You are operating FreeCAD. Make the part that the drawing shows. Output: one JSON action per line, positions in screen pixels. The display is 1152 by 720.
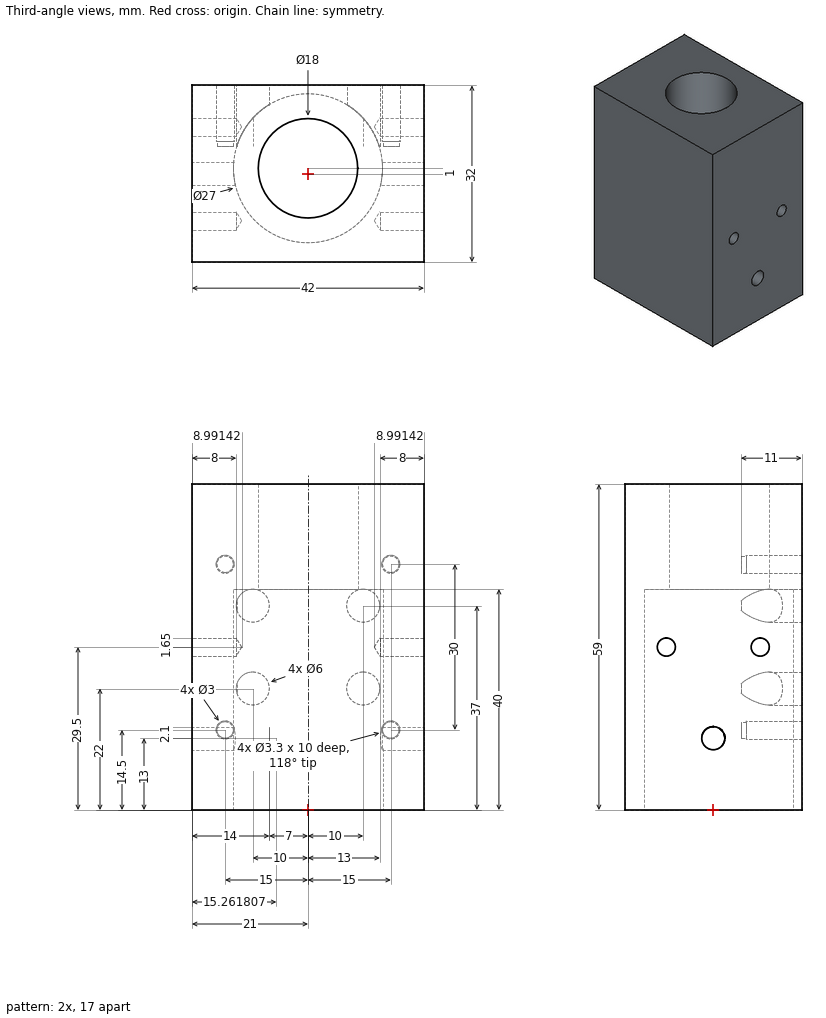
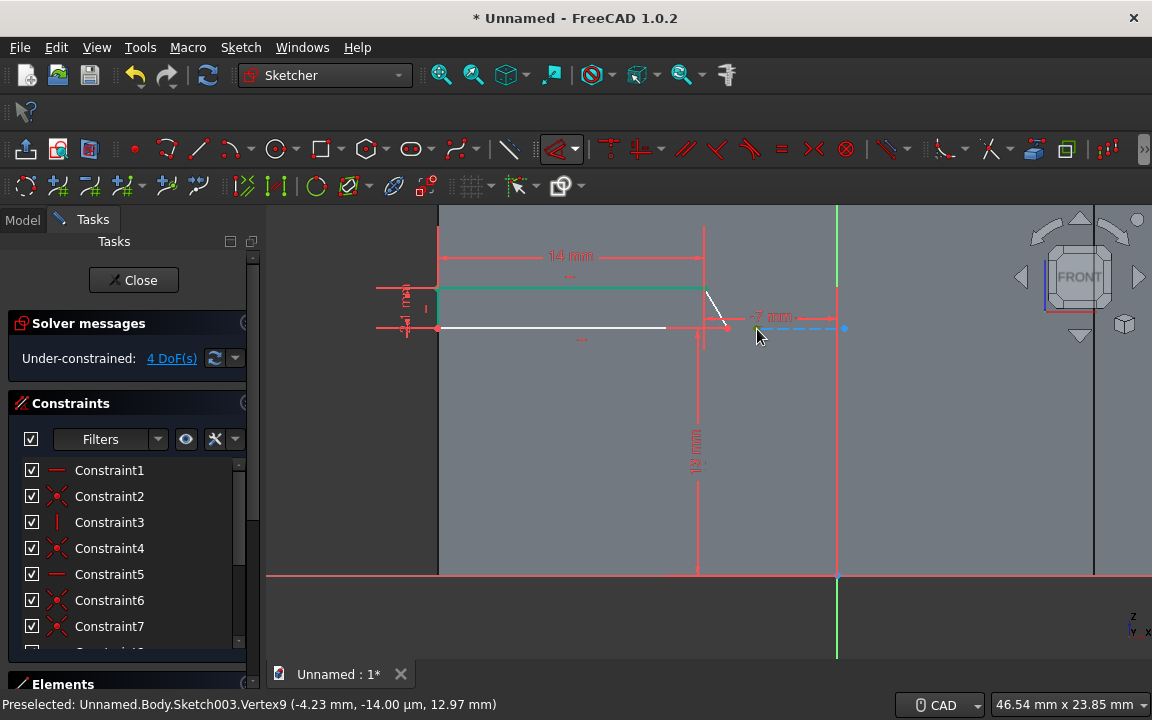
{"action": "key", "text": "i"}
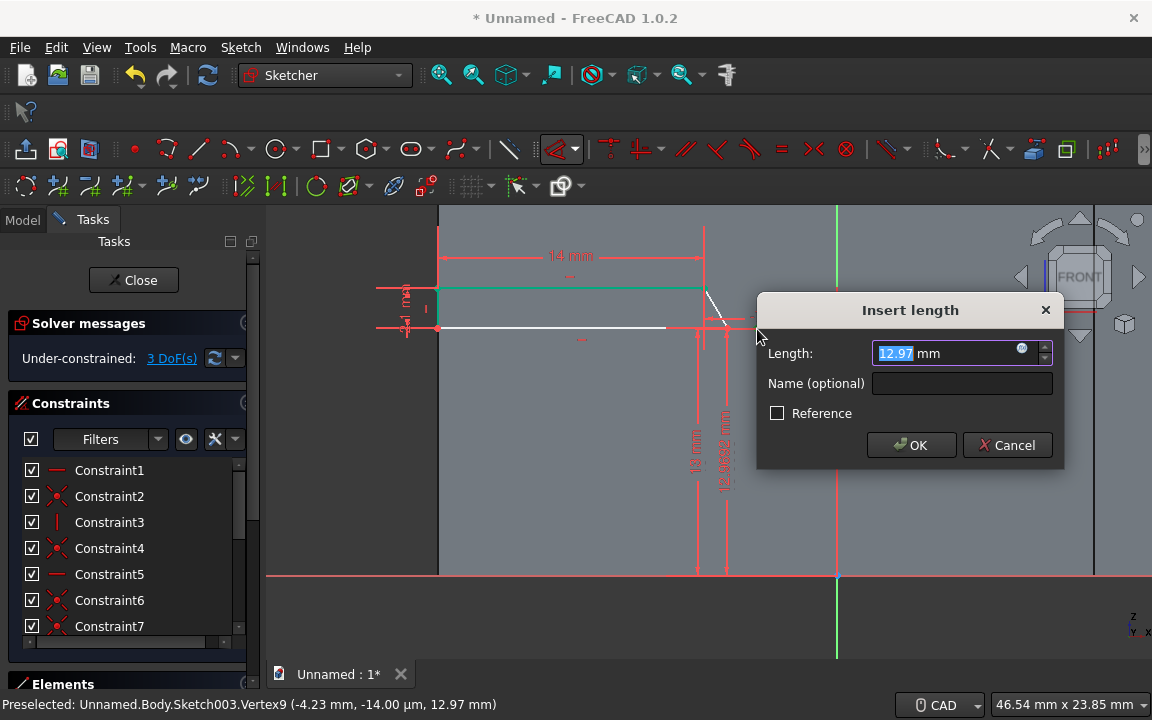
{"action": "type", "text": "13"}
{"action": "key", "text": "Return"}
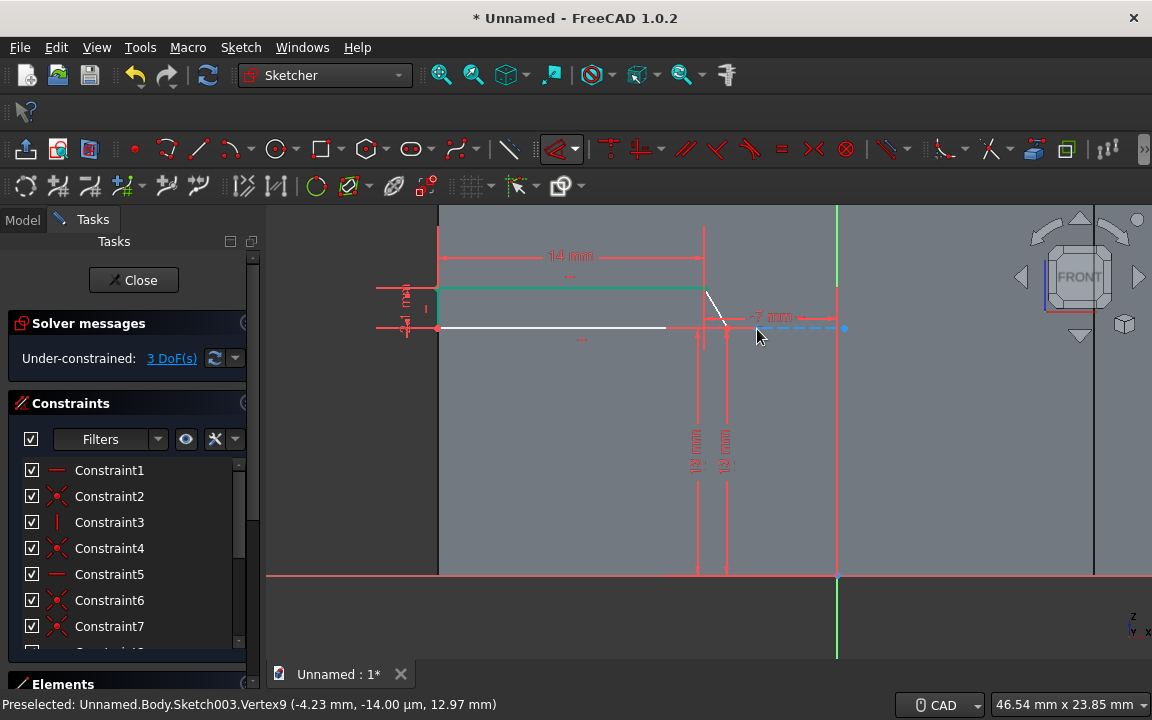
{"action": "left_click", "coordinate": [641, 328]}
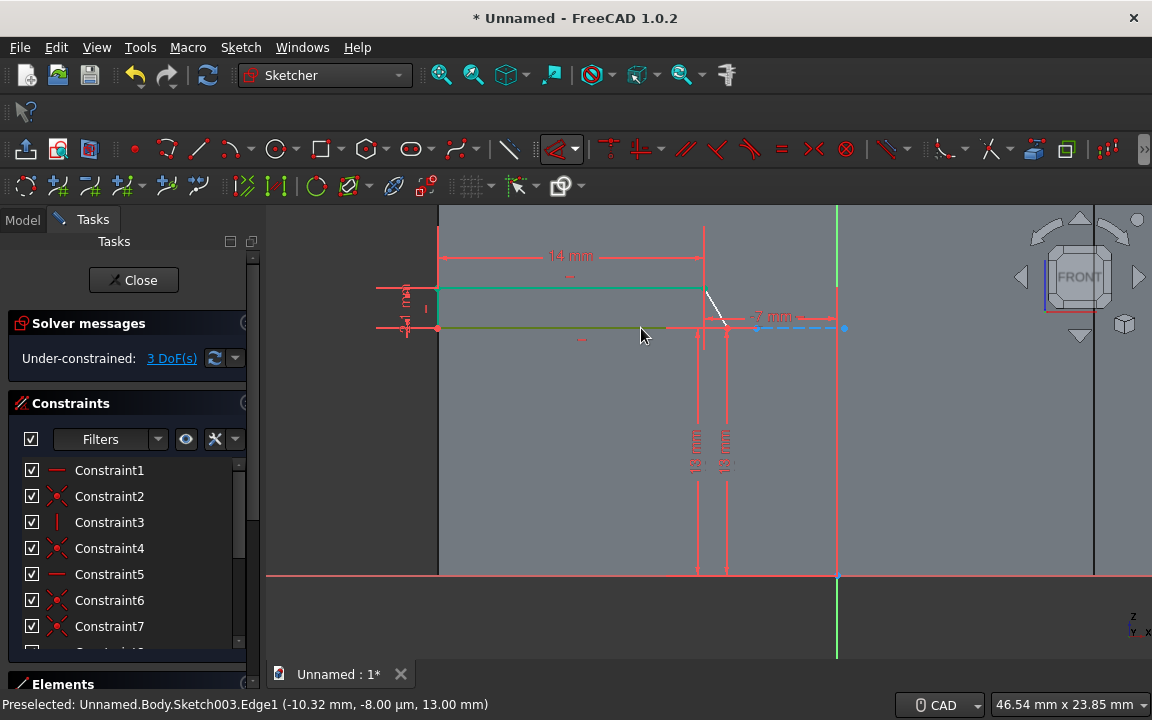
{"action": "key", "text": "l"}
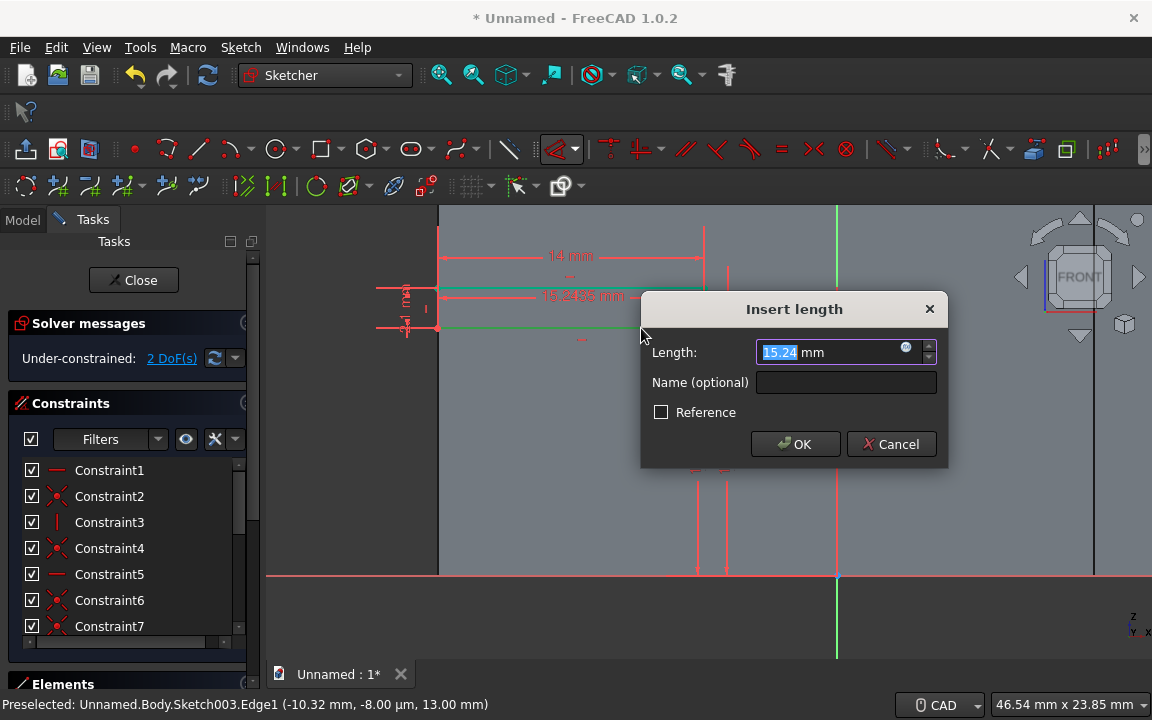
{"action": "type", "text": "15.261807"}
{"action": "key", "text": "Return"}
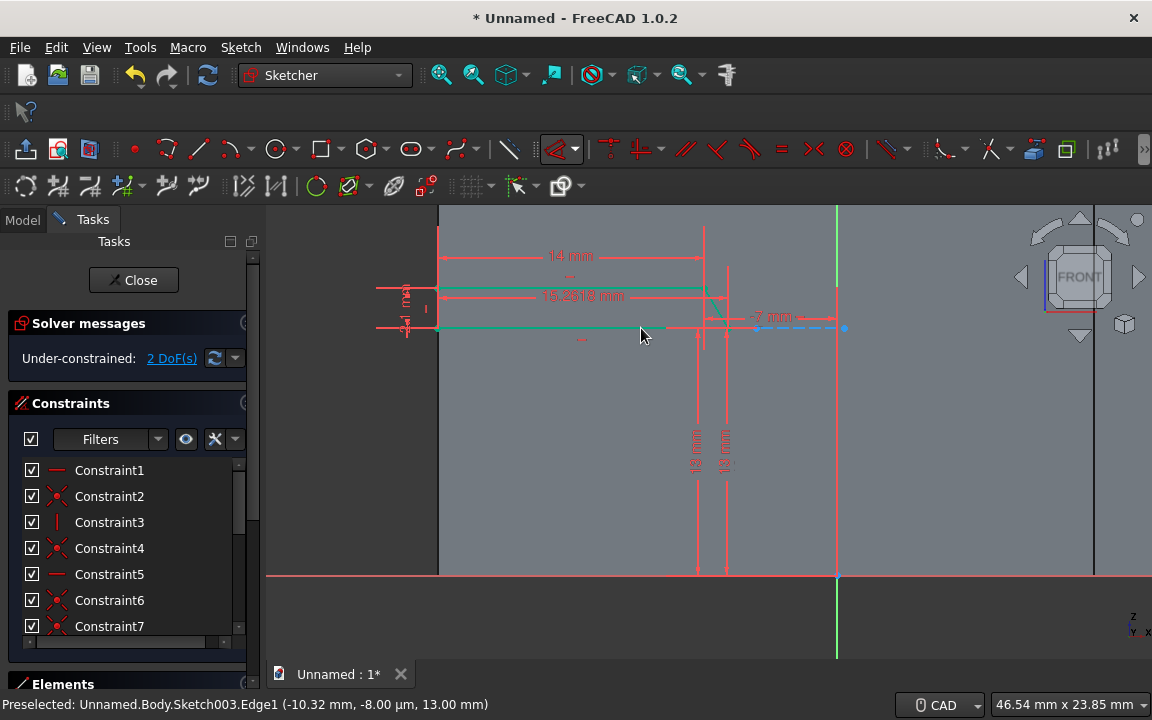
{"action": "left_click", "coordinate": [134, 280]}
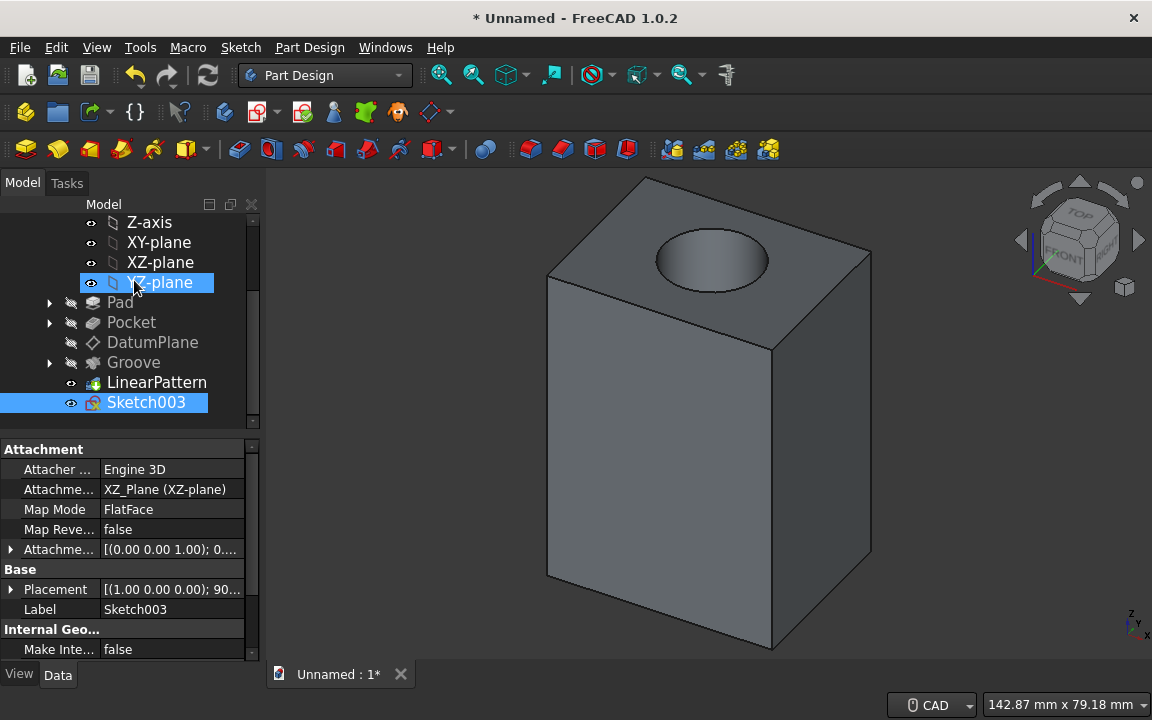
{"action": "left_click", "coordinate": [304, 150]}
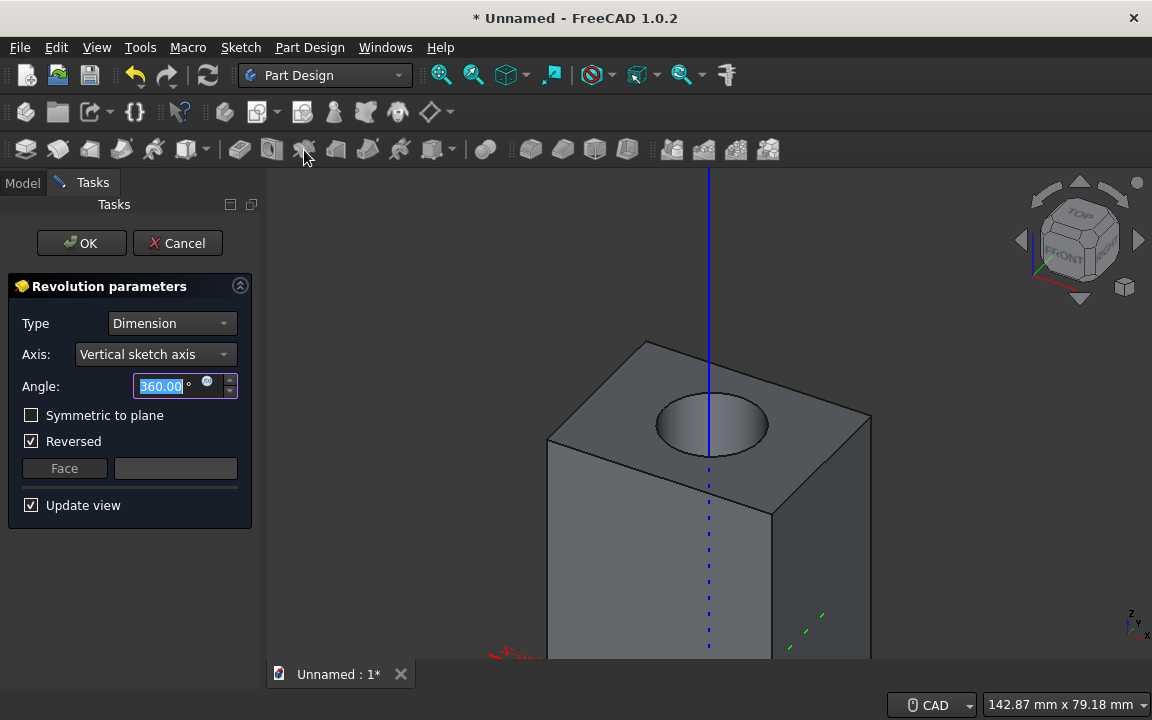
{"action": "left_click", "coordinate": [156, 354]}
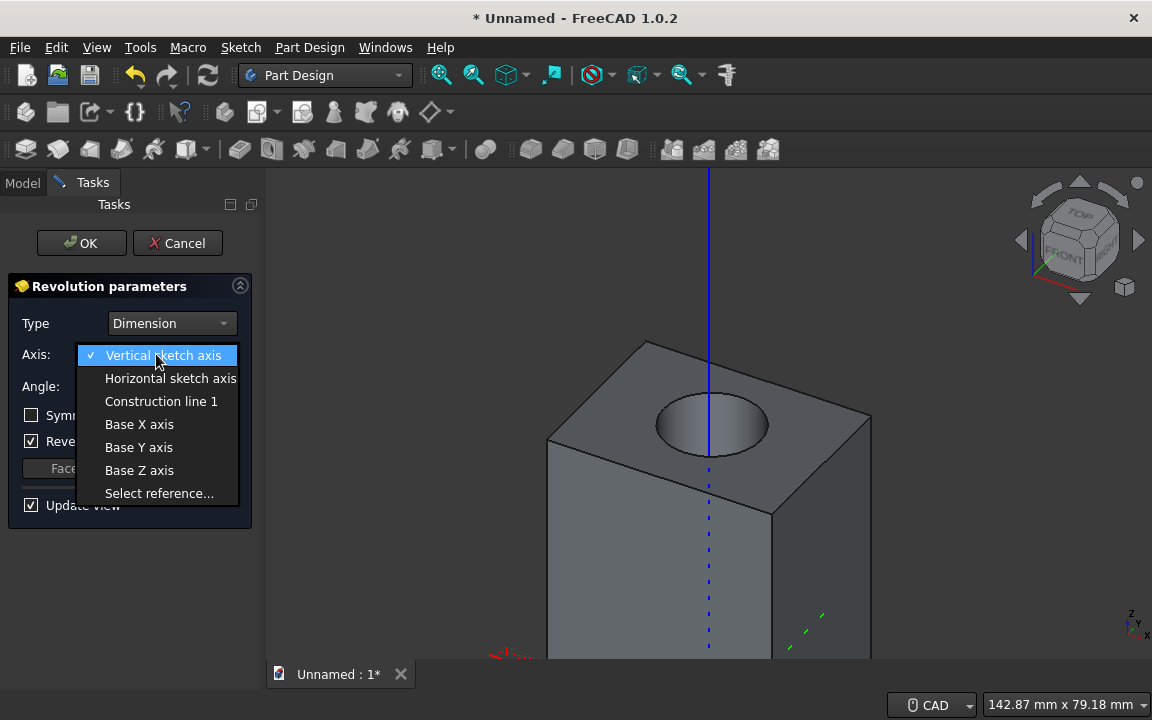
{"action": "left_click", "coordinate": [156, 402]}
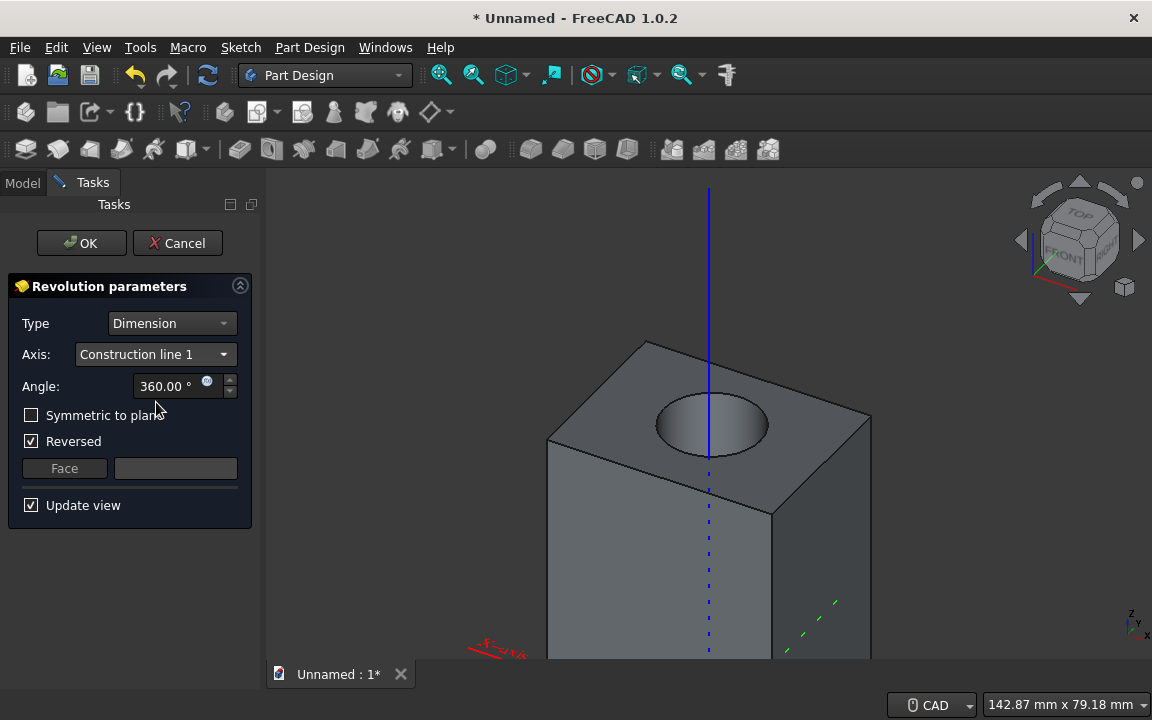
{"action": "left_click", "coordinate": [82, 243]}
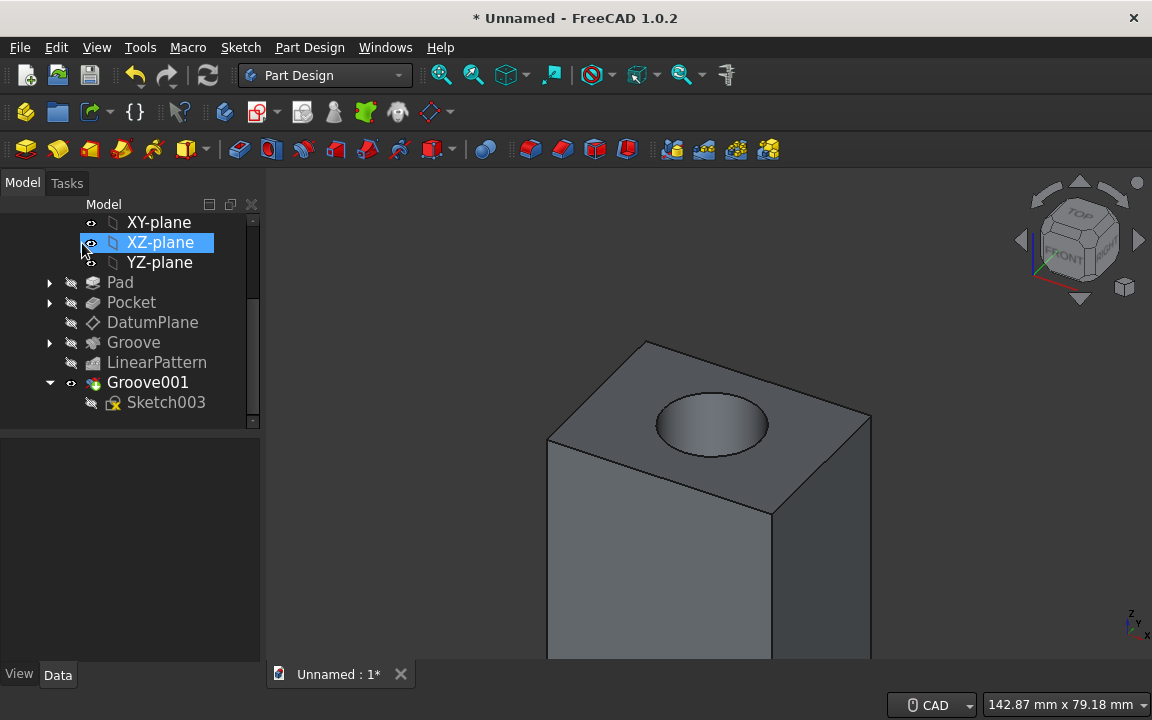
{"action": "key", "text": "v f"}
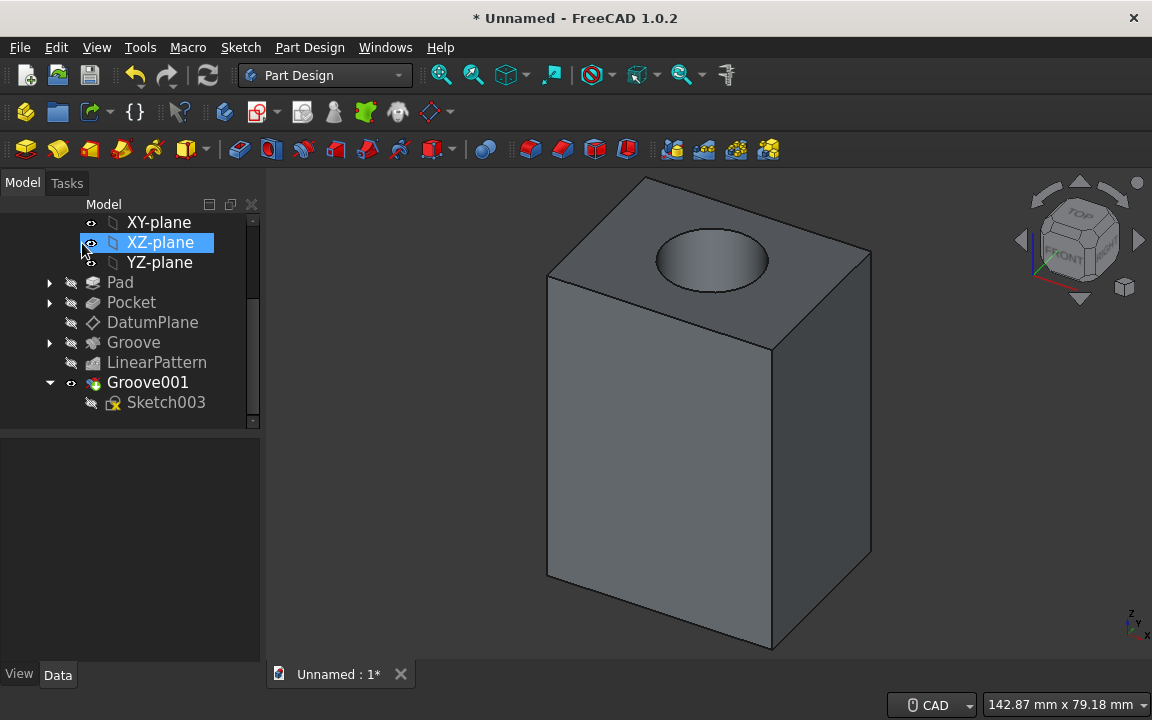
{"action": "left_click", "coordinate": [116, 343]}